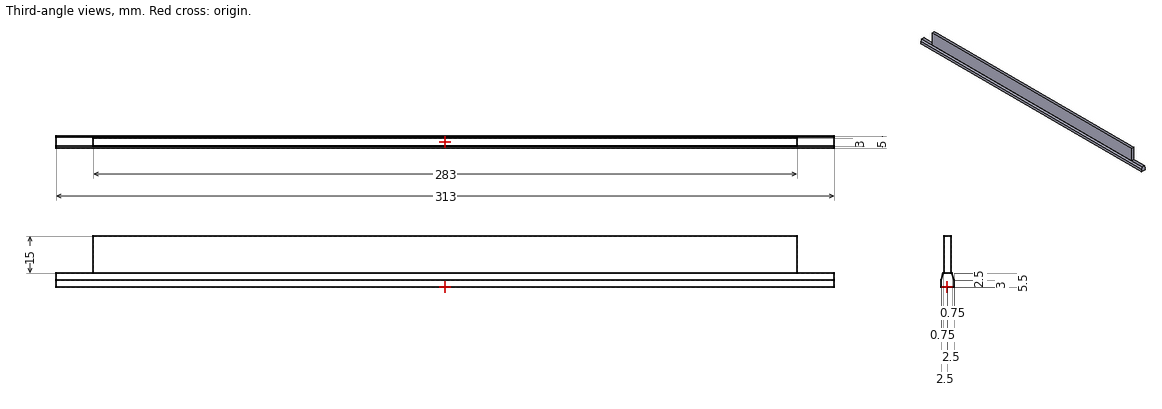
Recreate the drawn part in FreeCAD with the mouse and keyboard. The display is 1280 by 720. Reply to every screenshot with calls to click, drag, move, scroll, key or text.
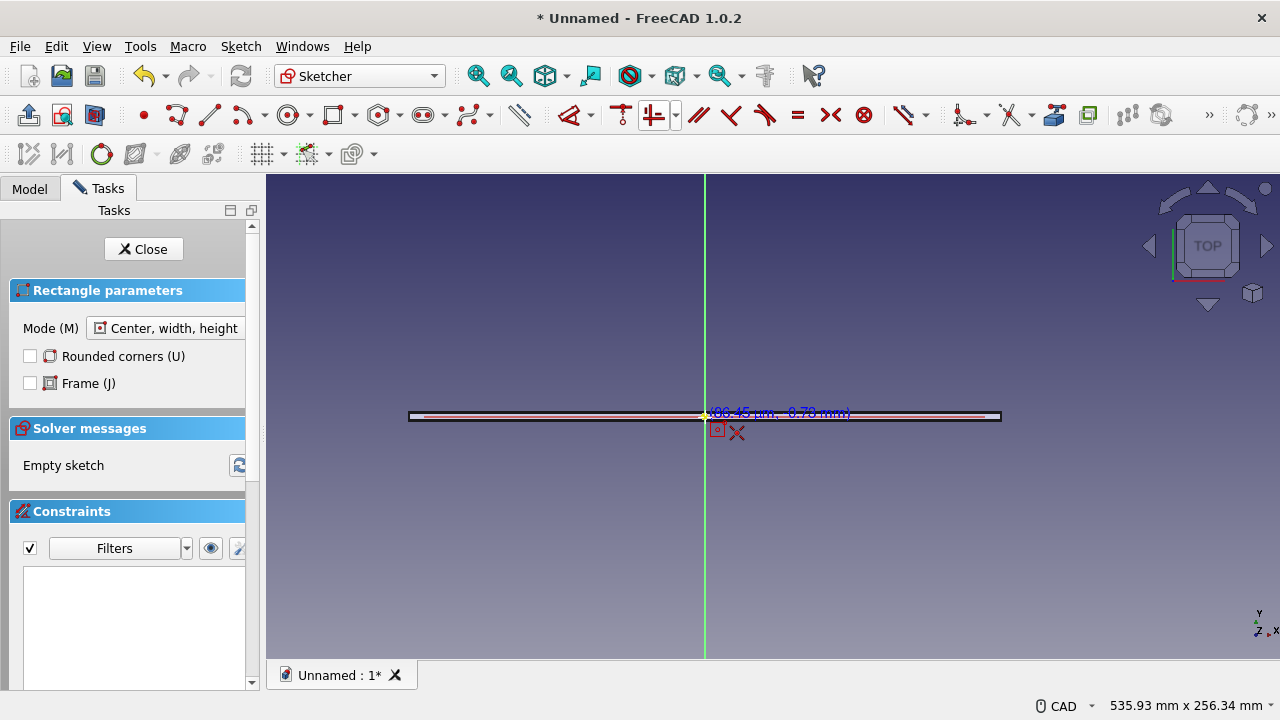
click(705, 417)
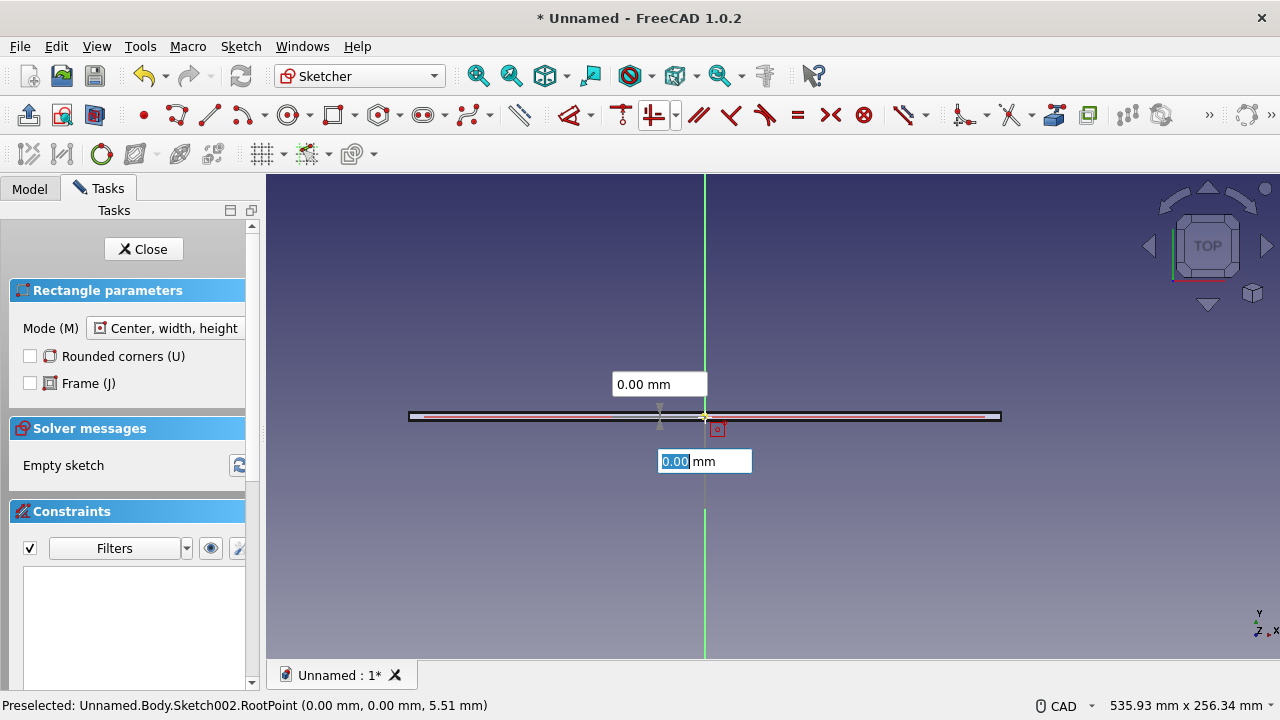
scroll(973, 414, up, 9)
move(967, 410)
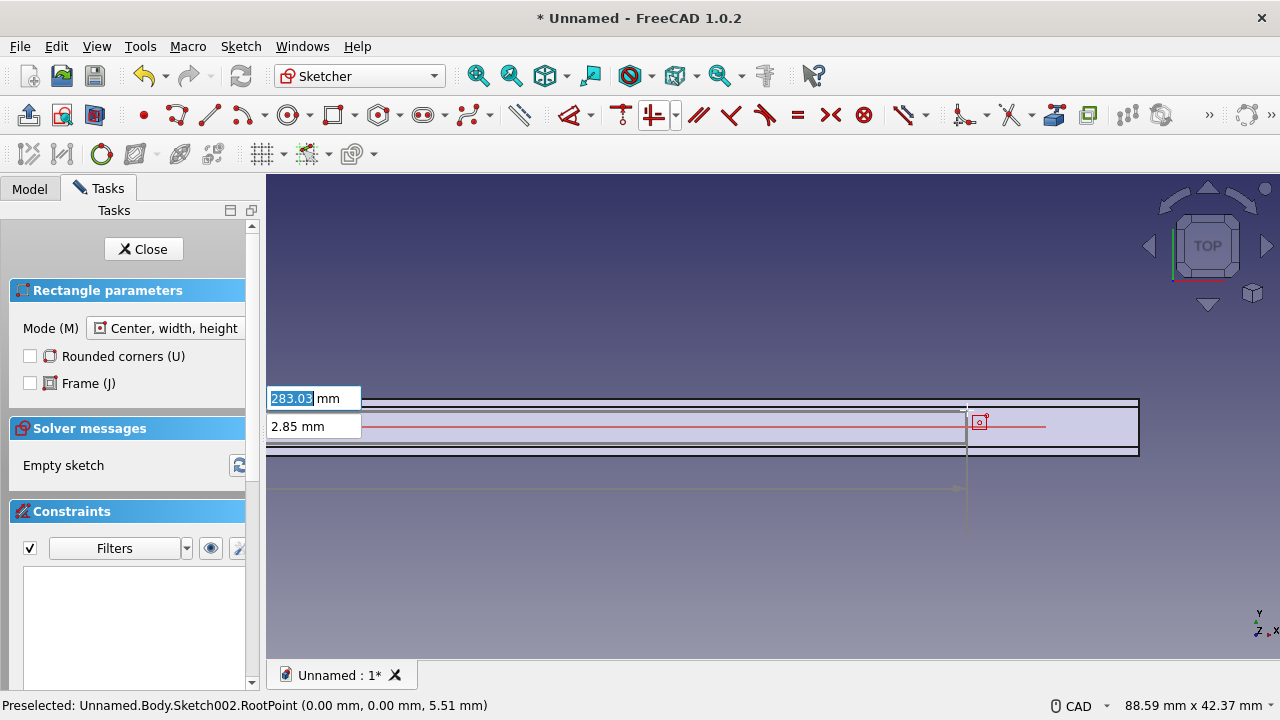
text(283)
key(Tab)
text(3)
key(Return)
key(Escape)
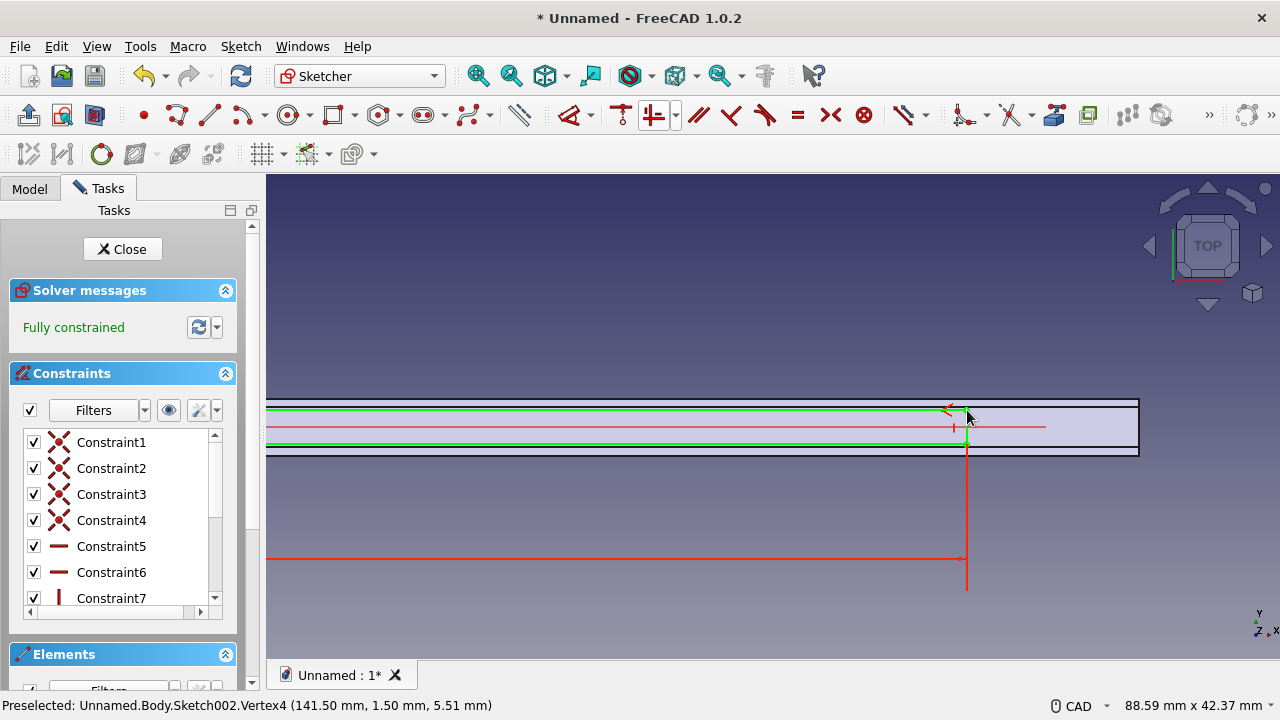
click(123, 249)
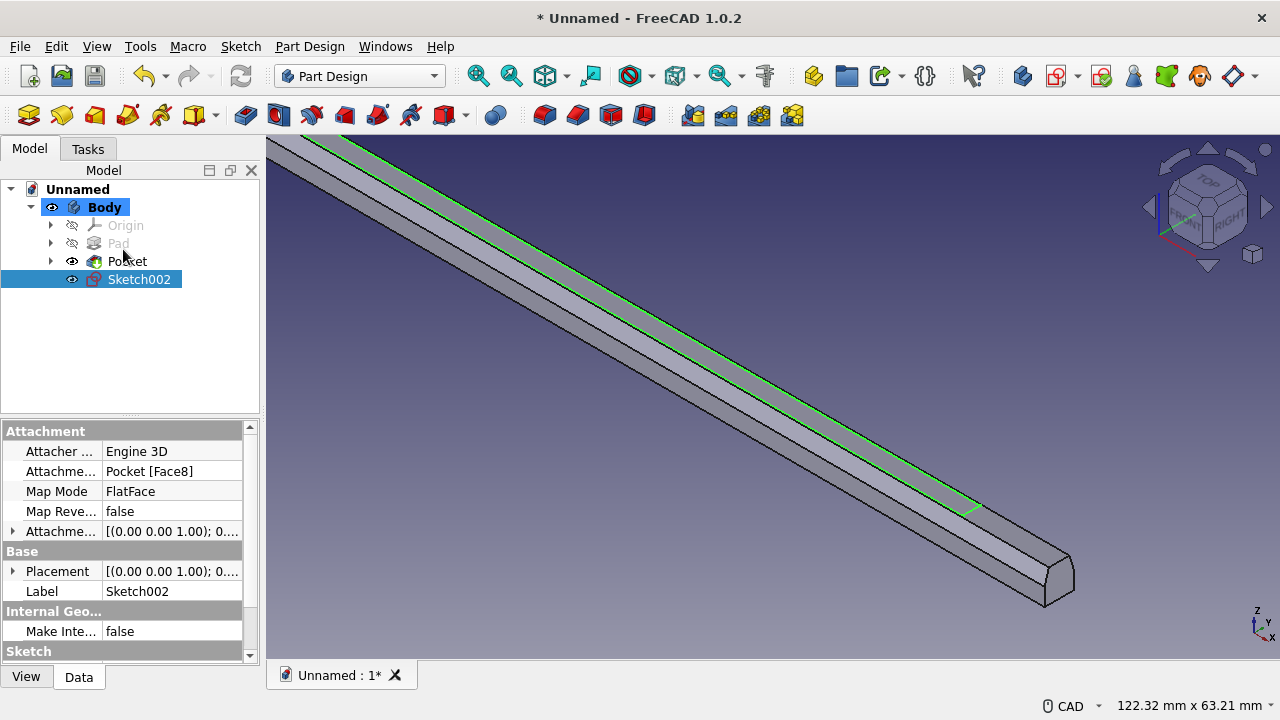
click(29, 116)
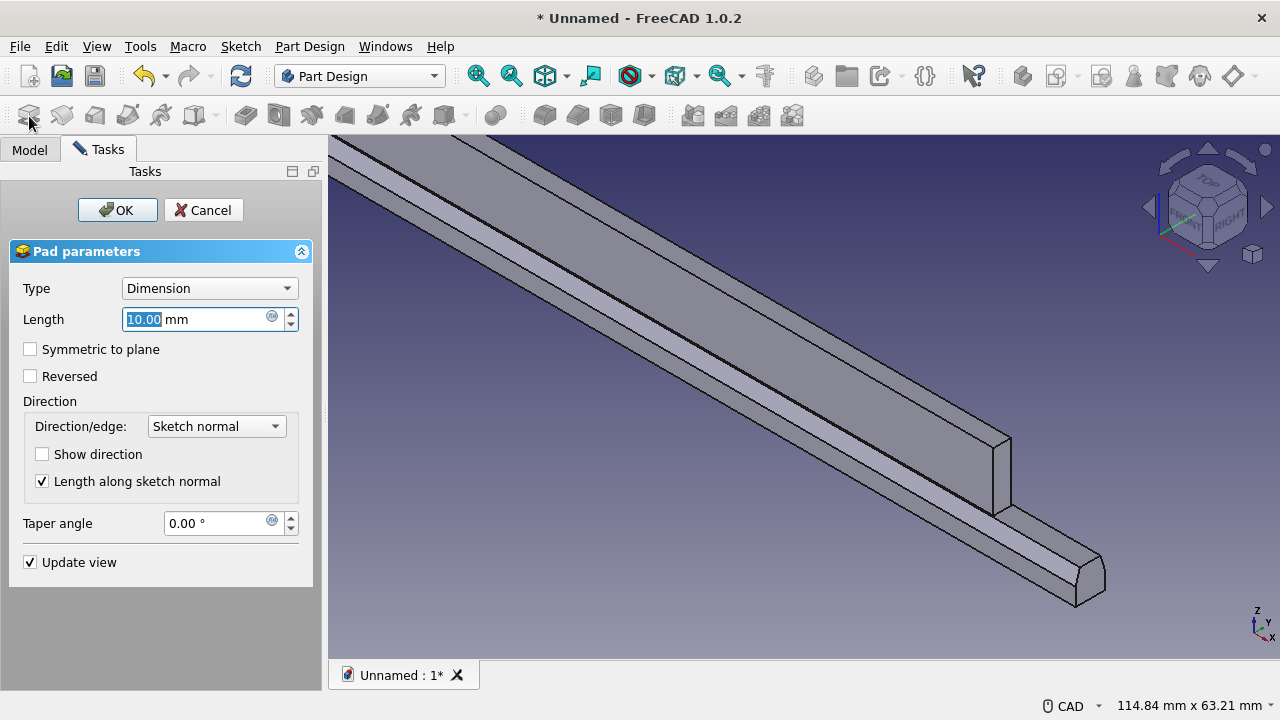
text(15)
key(Tab)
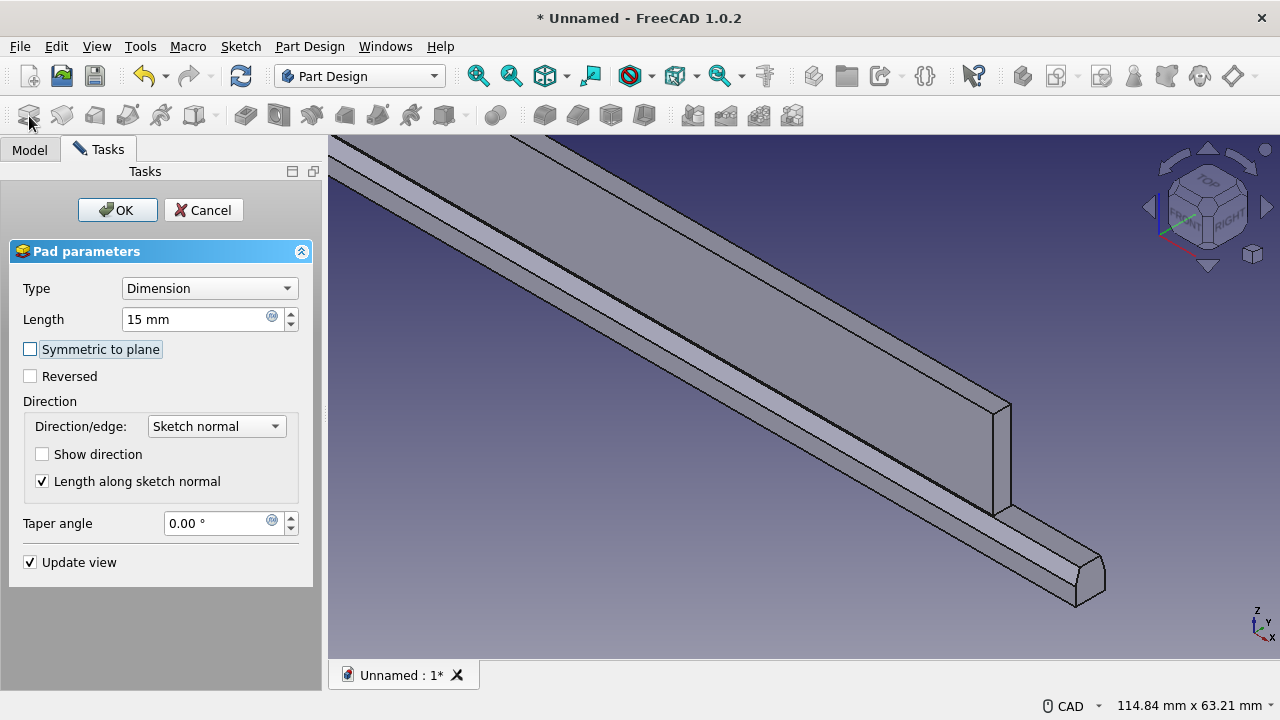
click(118, 210)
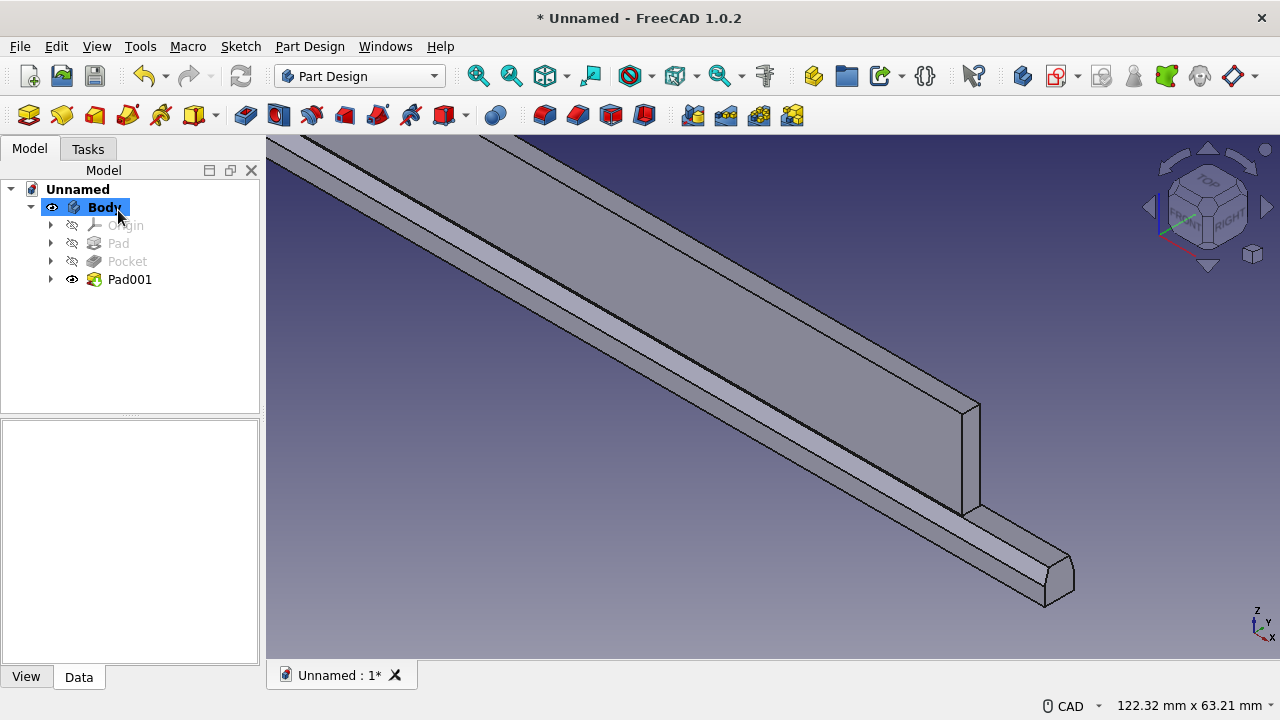
click(479, 76)